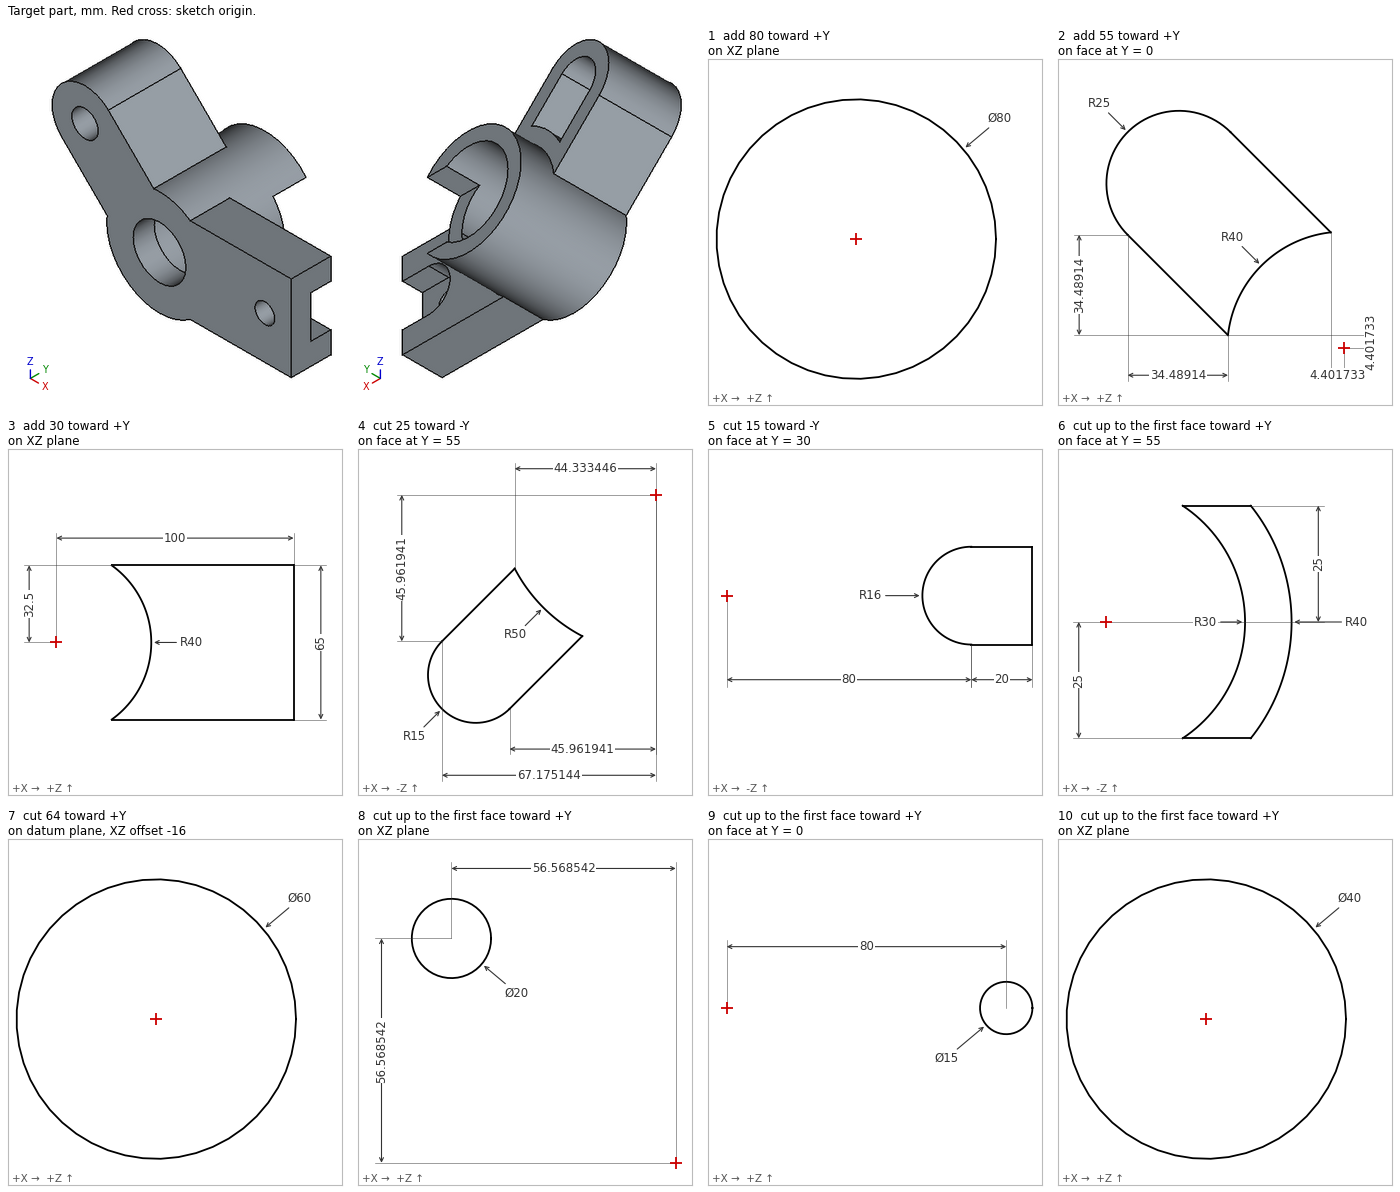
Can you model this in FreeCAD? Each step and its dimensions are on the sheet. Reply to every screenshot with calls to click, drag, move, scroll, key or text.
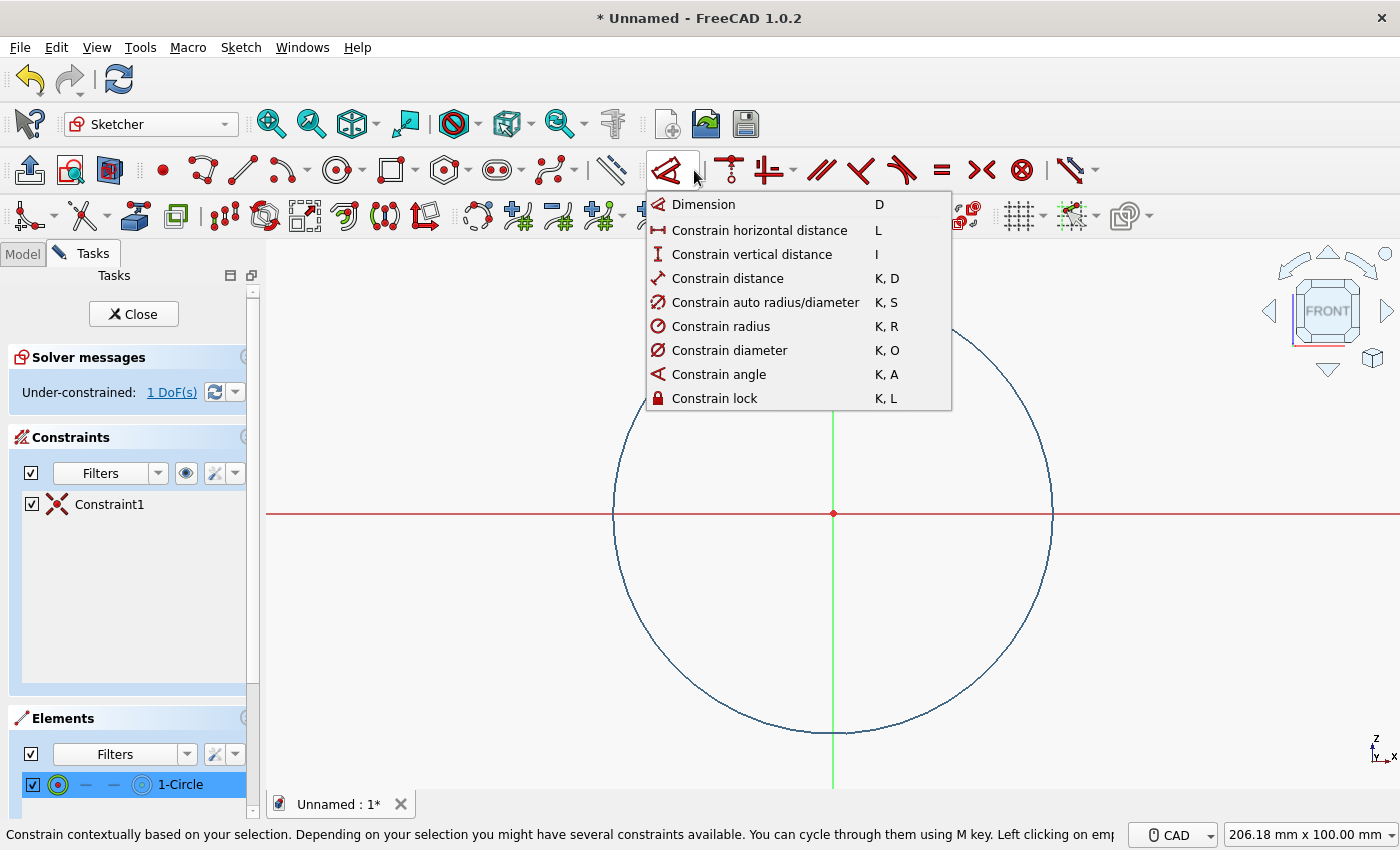
click(799, 350)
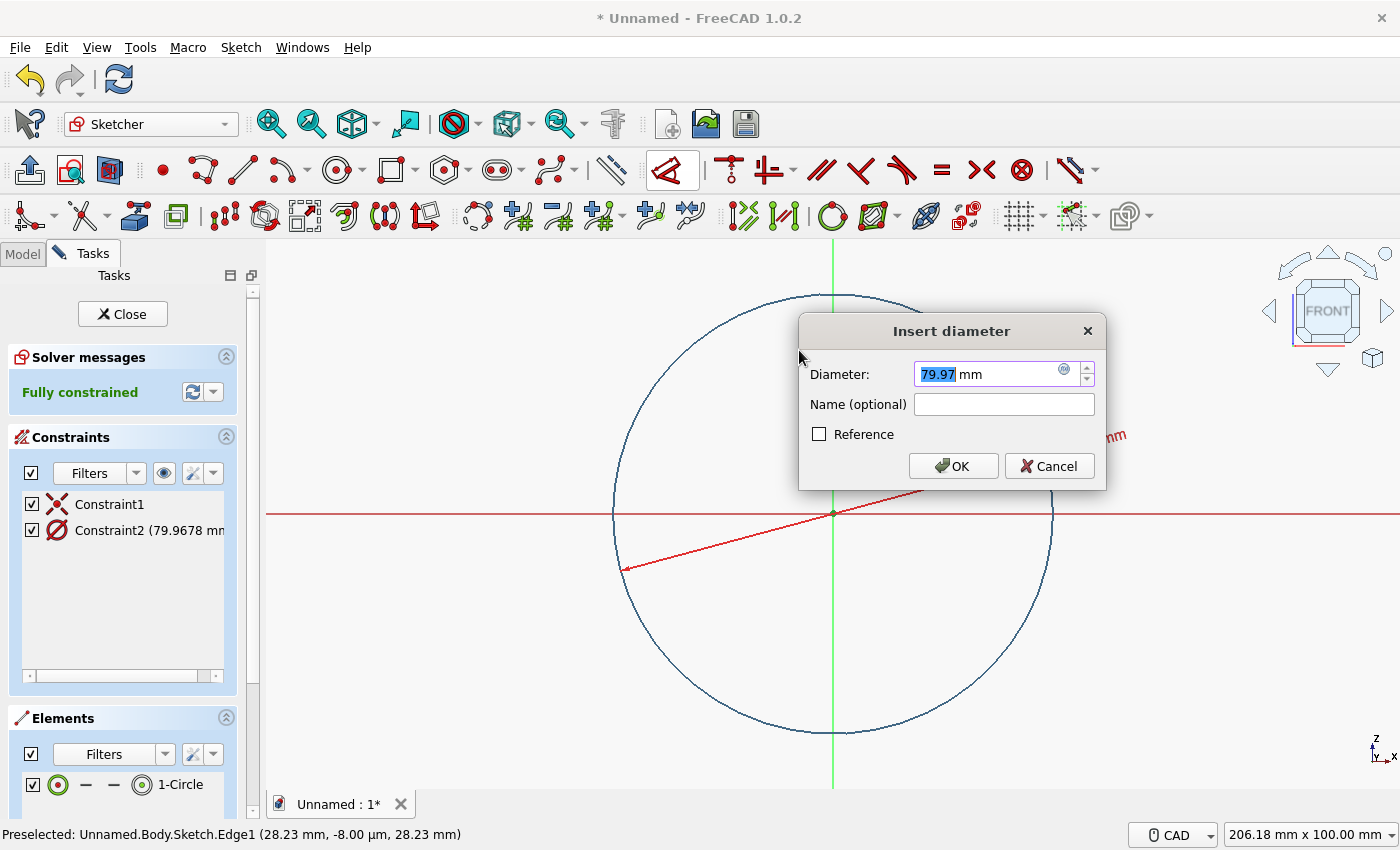
text(80)
key(Return)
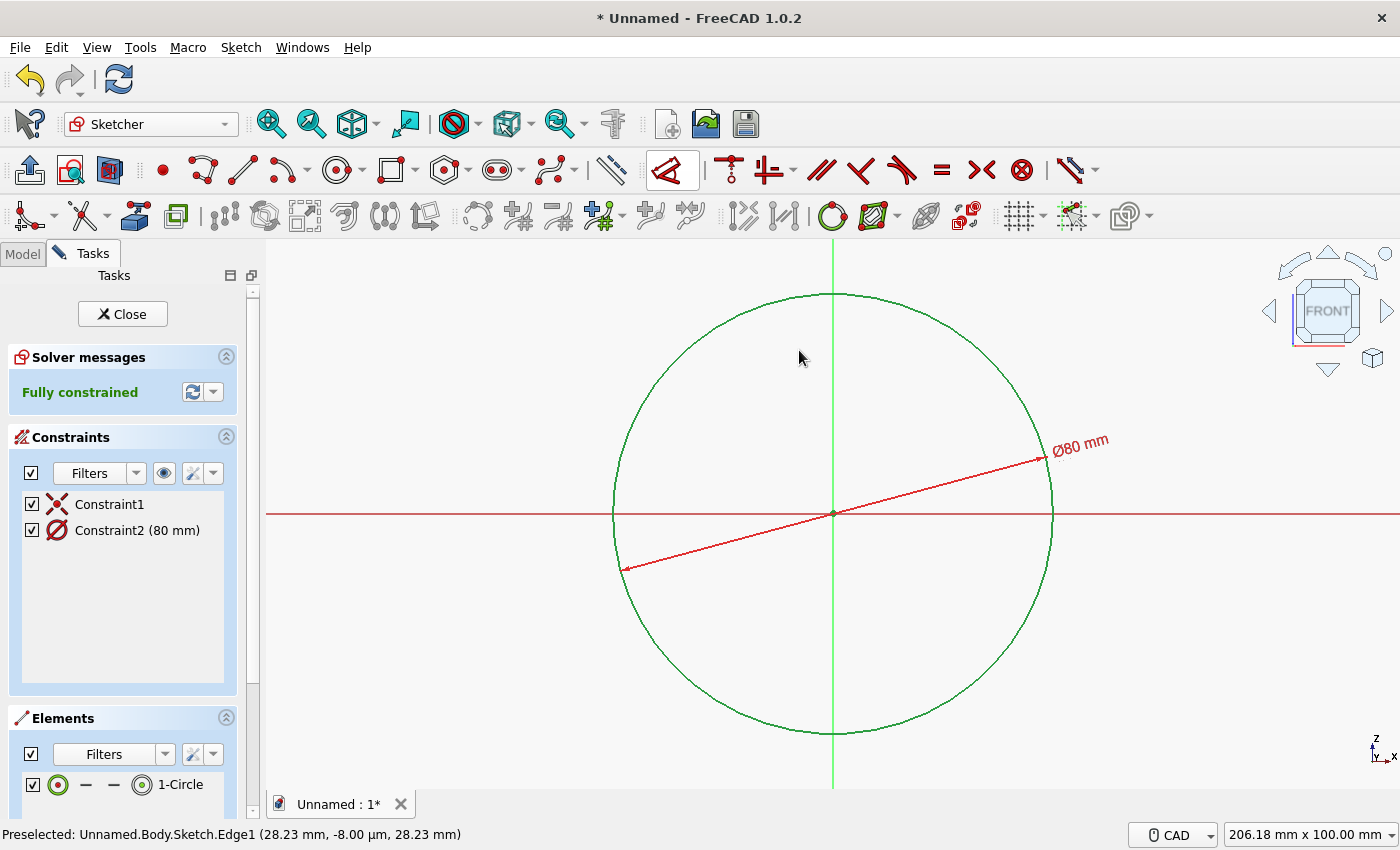
click(123, 314)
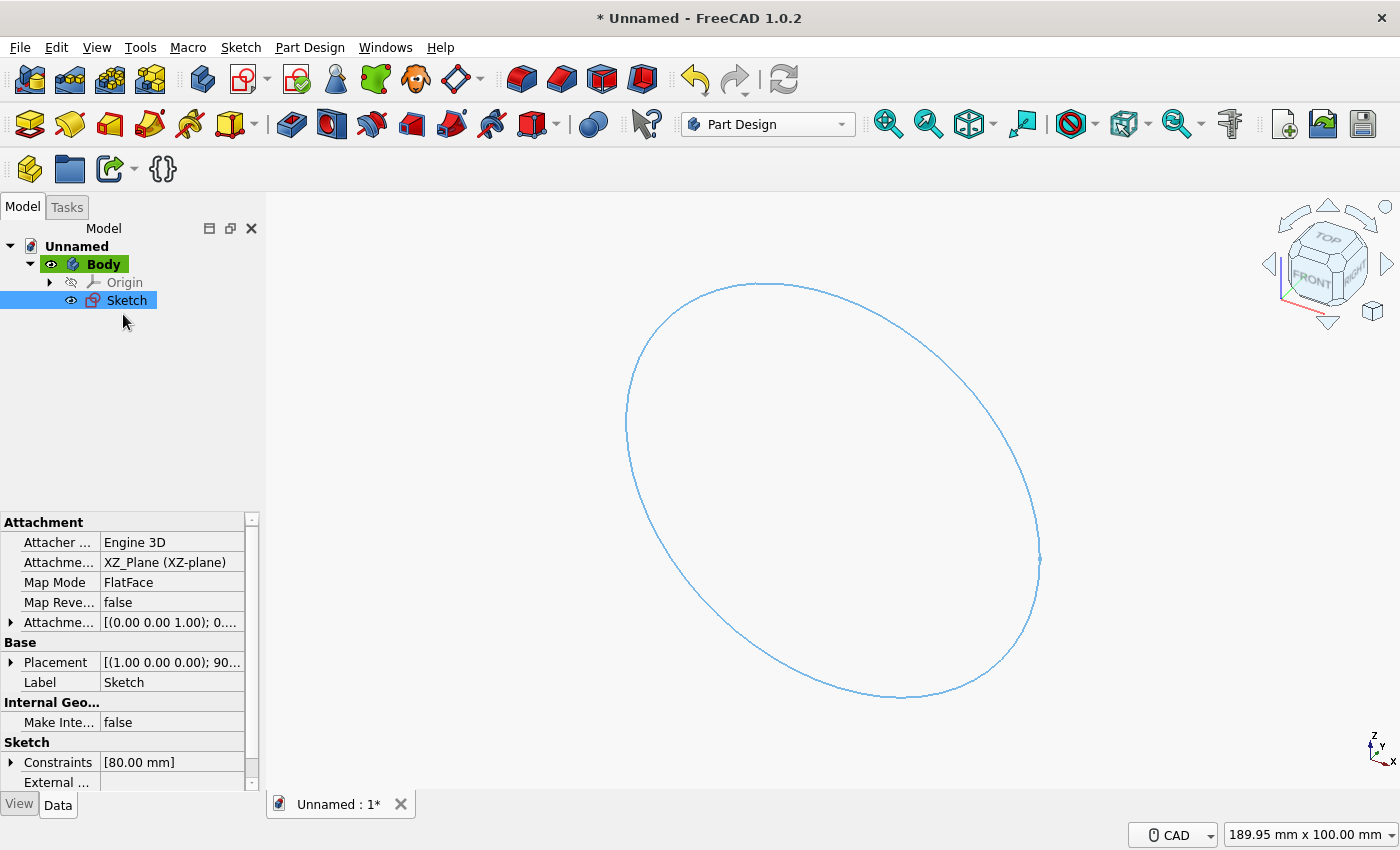
click(30, 124)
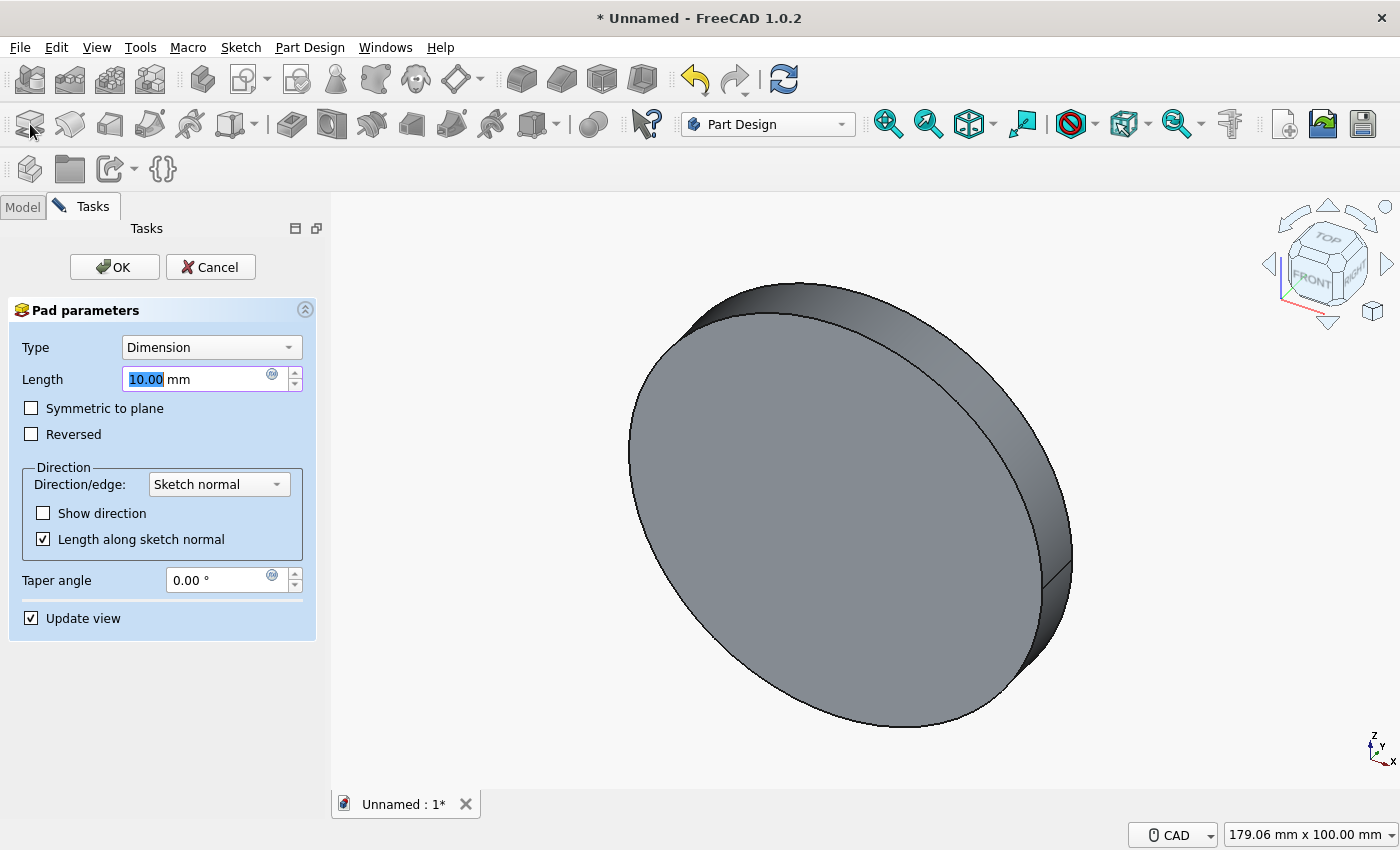
text(80)
key(Tab)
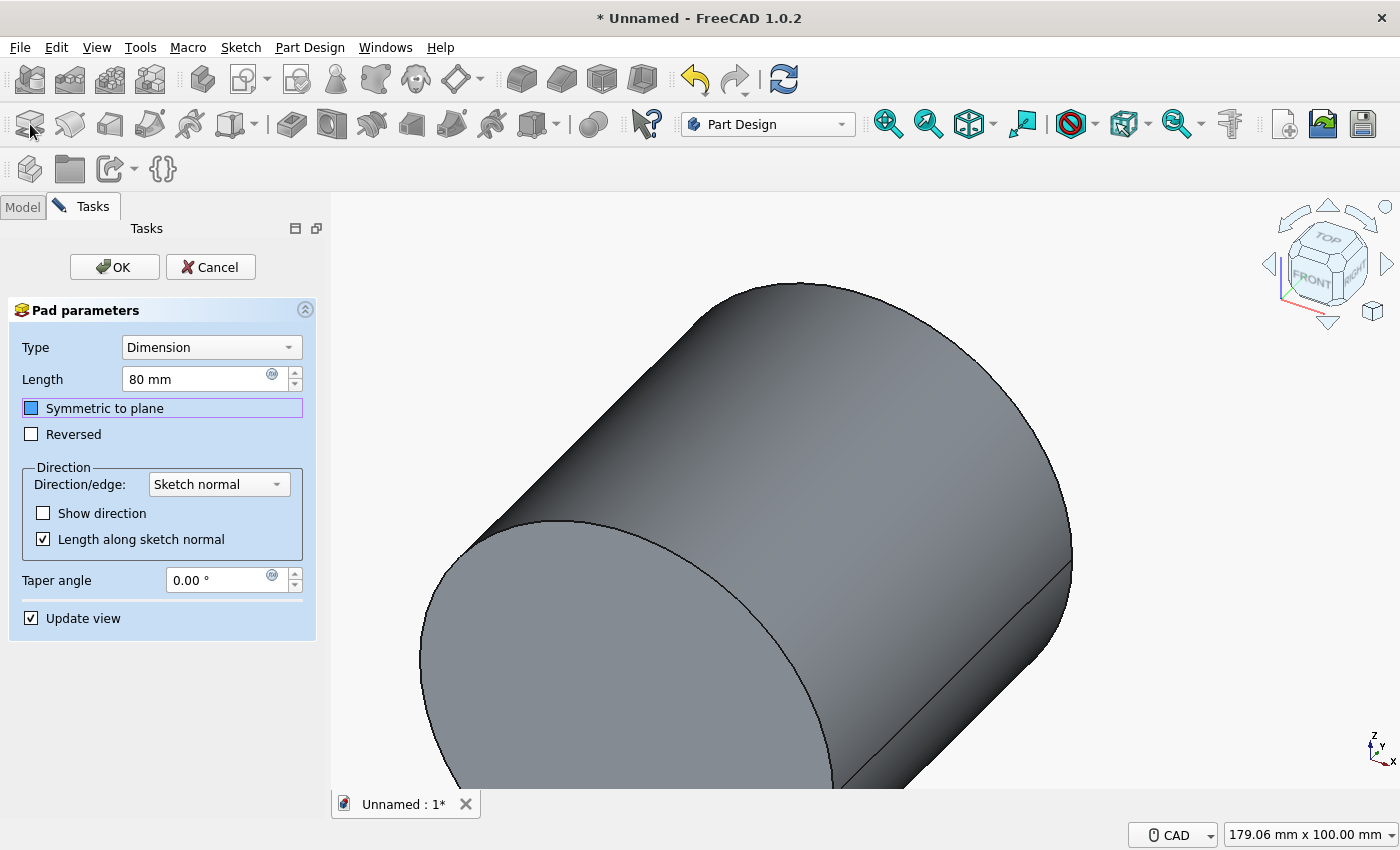
click(30, 434)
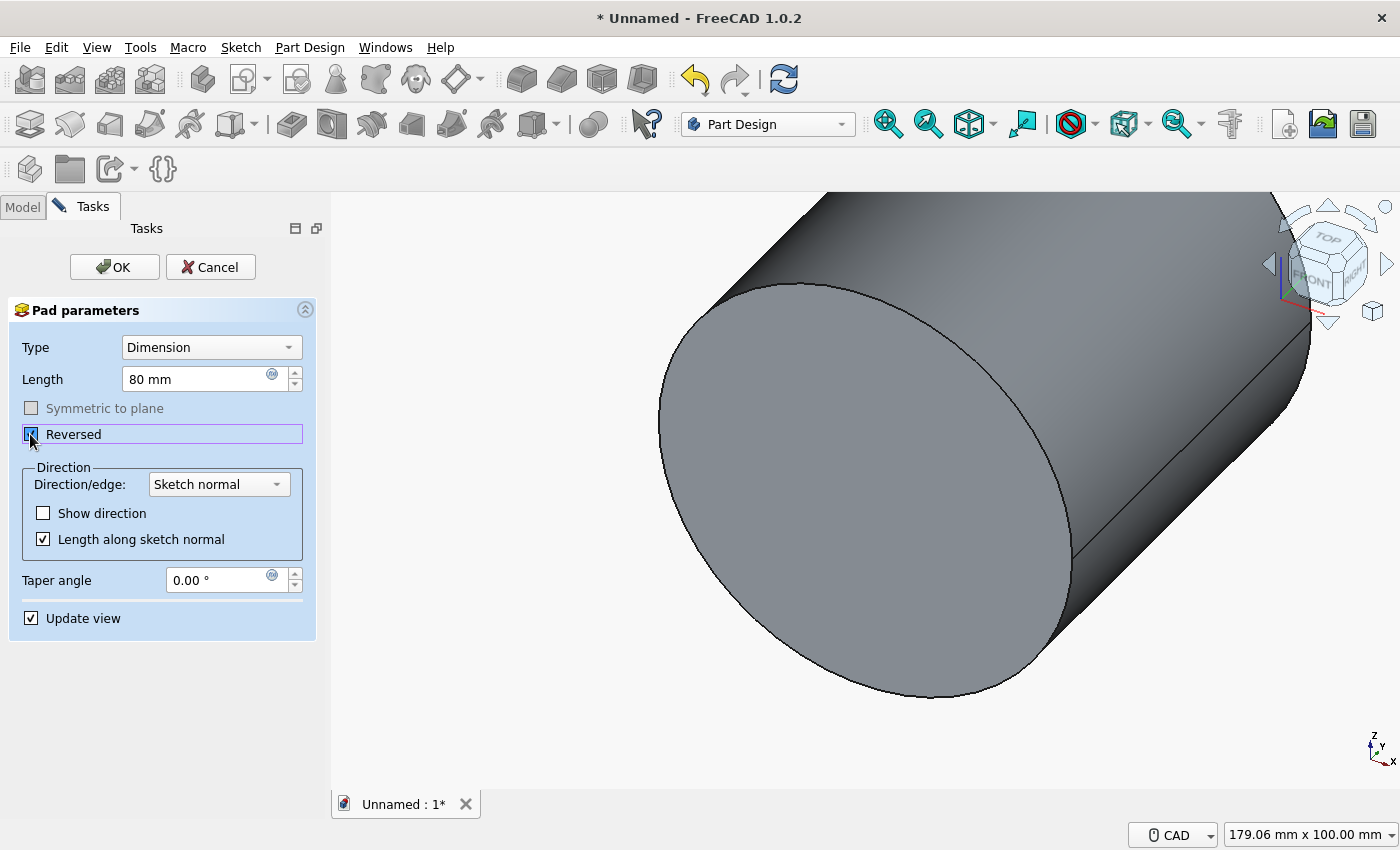
click(115, 267)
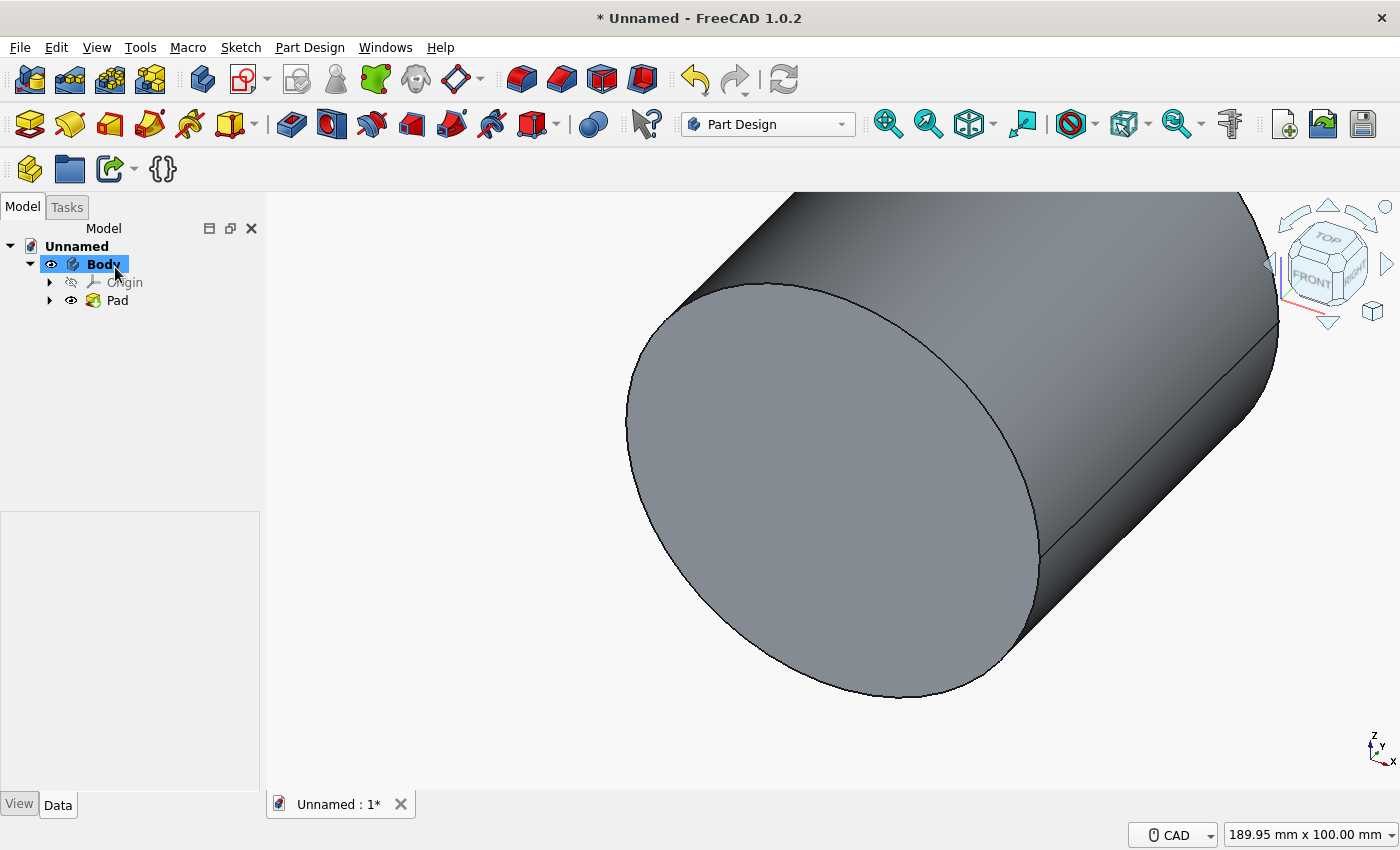
click(890, 124)